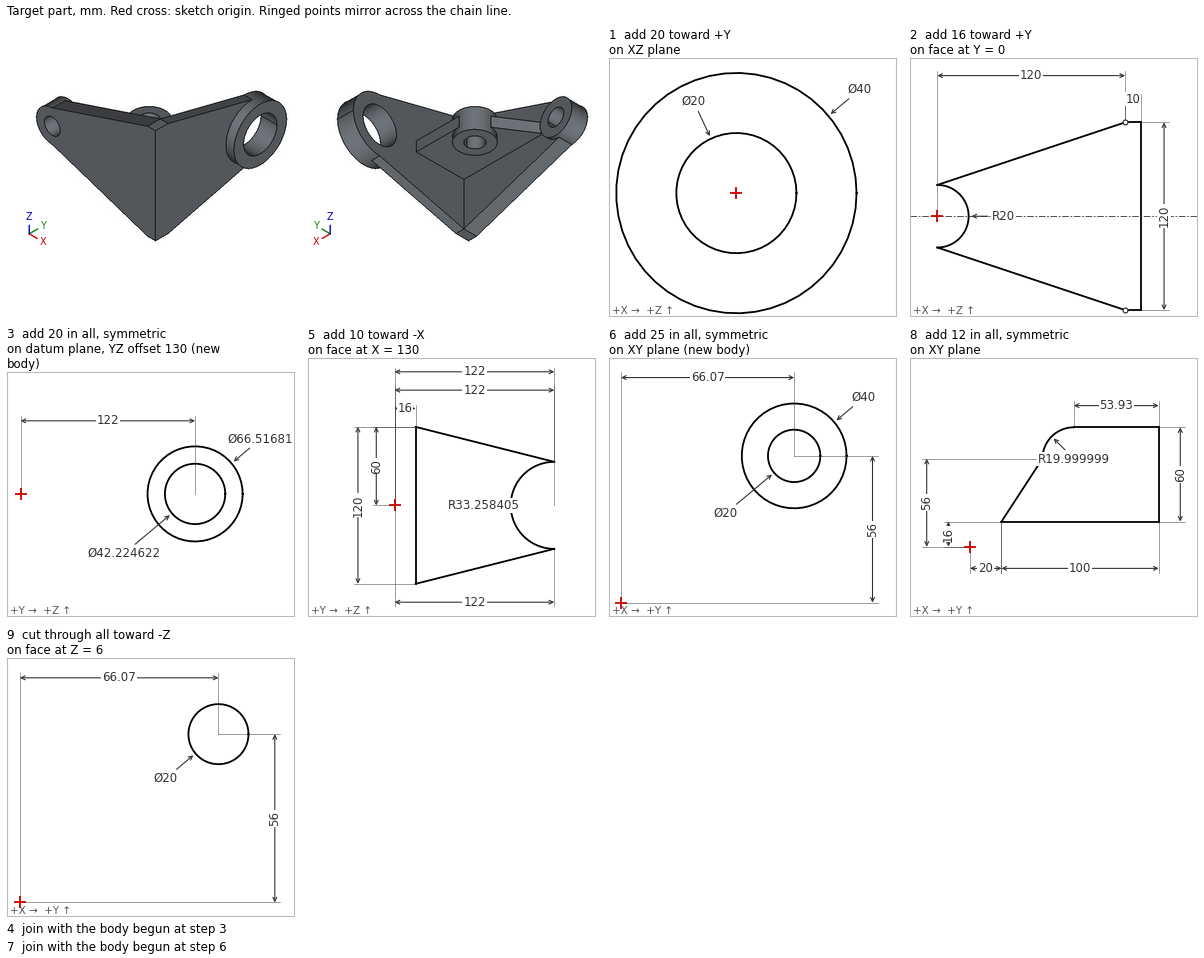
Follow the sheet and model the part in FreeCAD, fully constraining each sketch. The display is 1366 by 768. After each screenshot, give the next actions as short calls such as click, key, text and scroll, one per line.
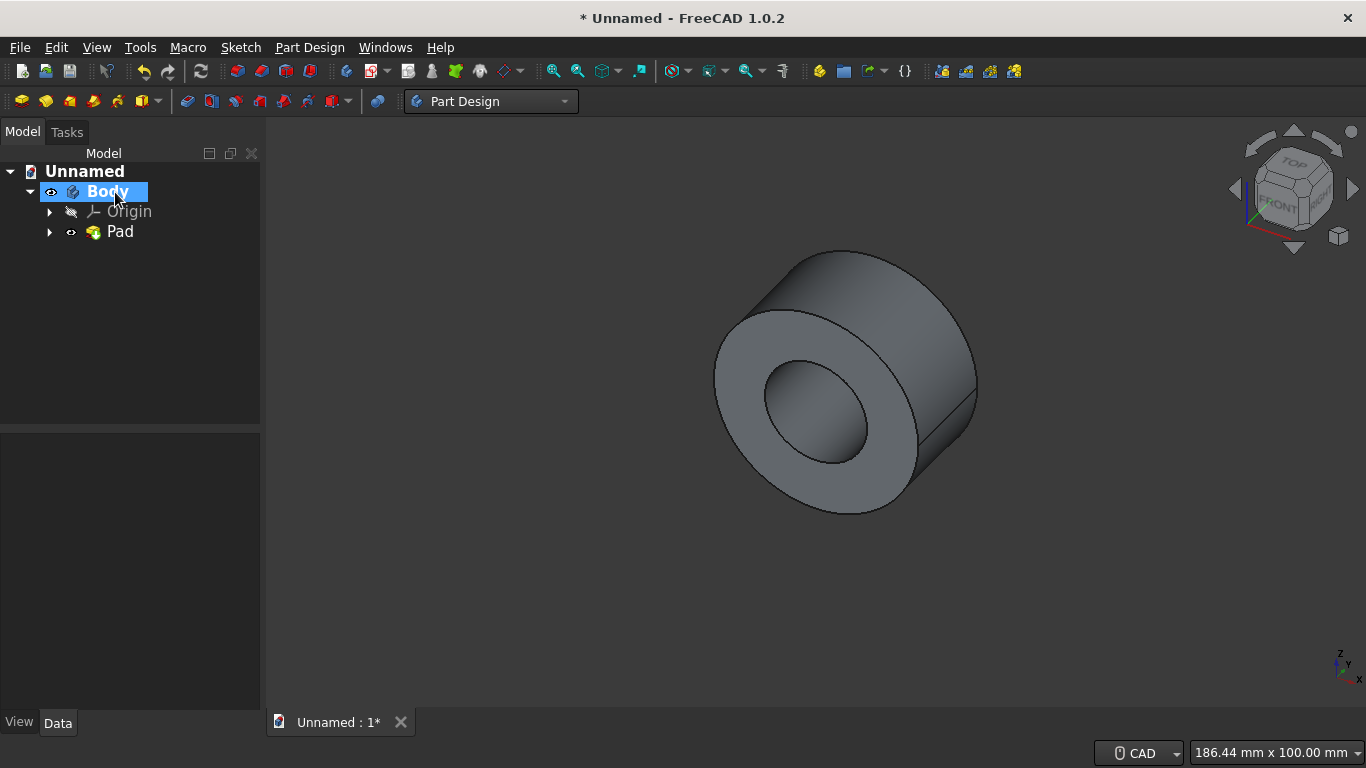
click(874, 486)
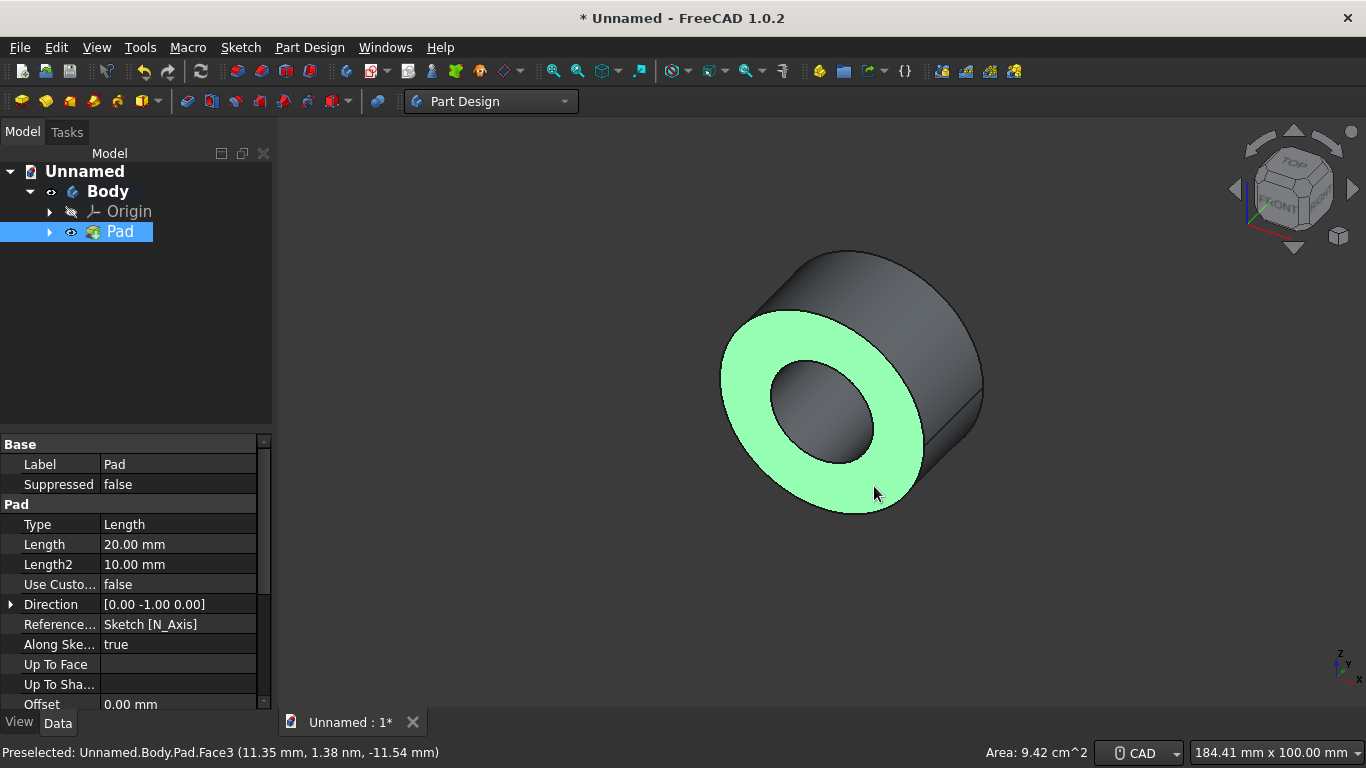
click(372, 72)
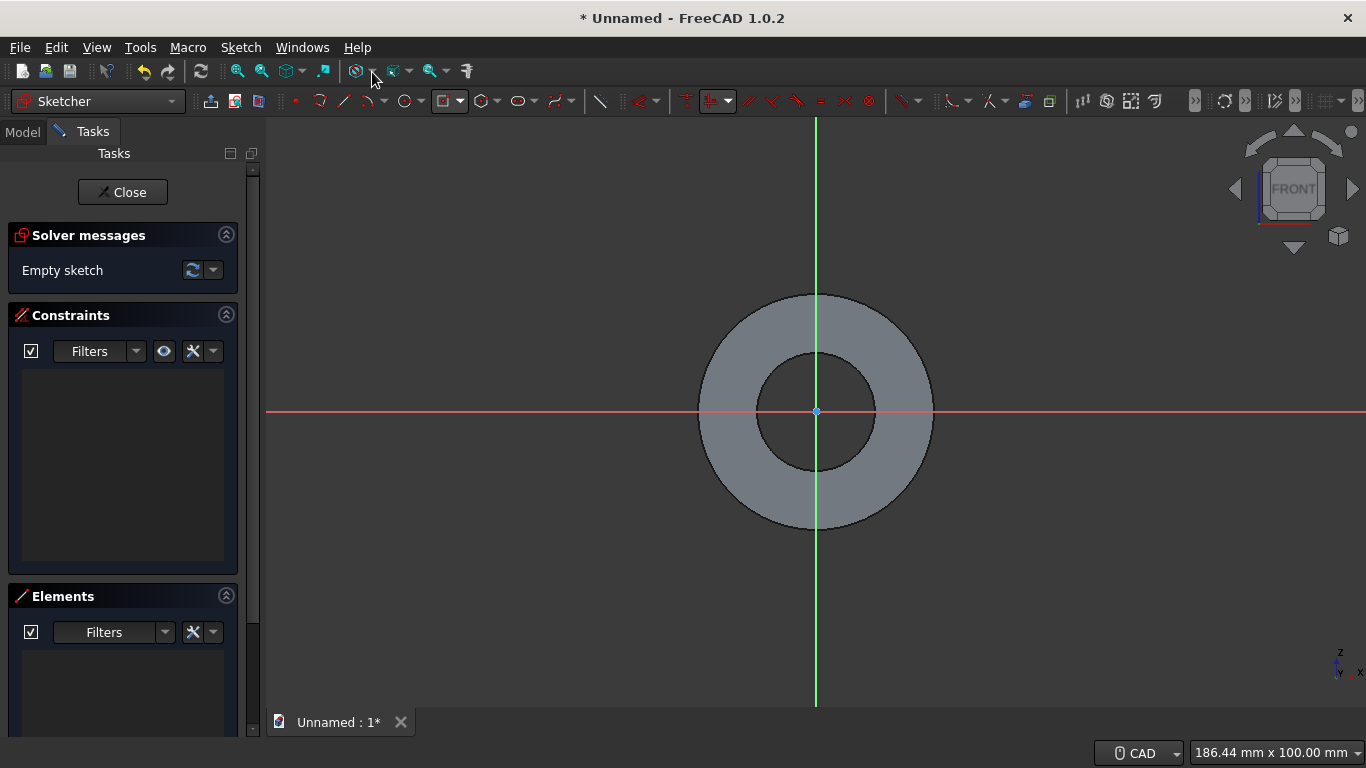
scroll(294, 412, down, 3)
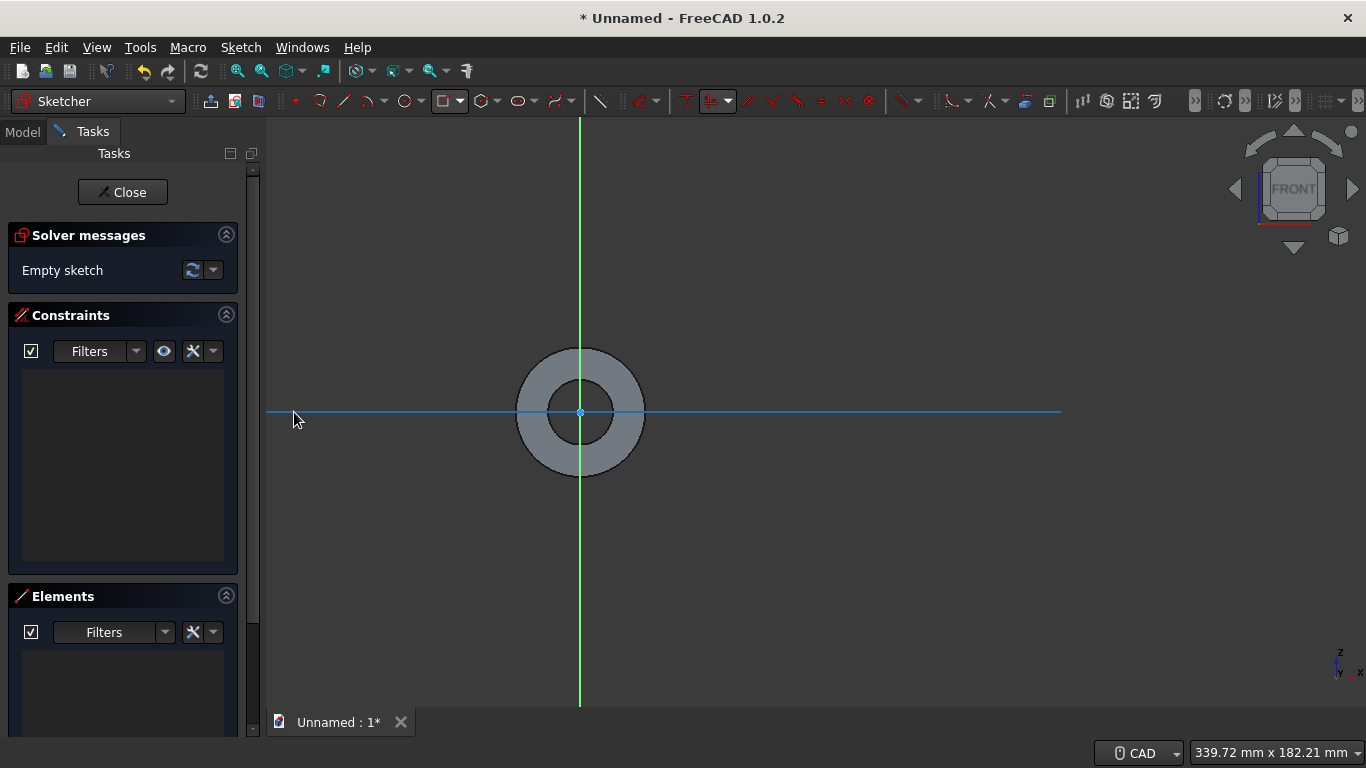
click(320, 102)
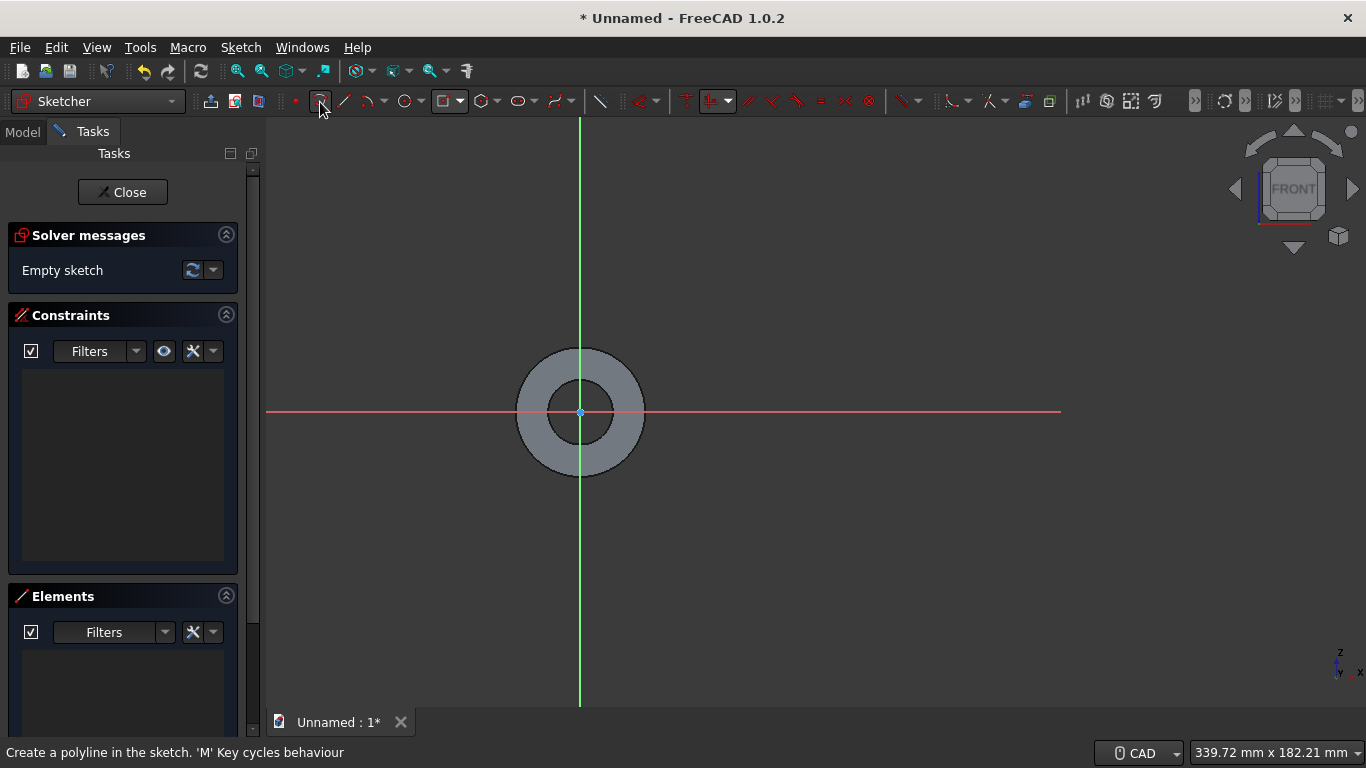
click(580, 347)
click(969, 218)
click(1001, 218)
click(1001, 607)
click(969, 607)
click(580, 477)
right_click(580, 477)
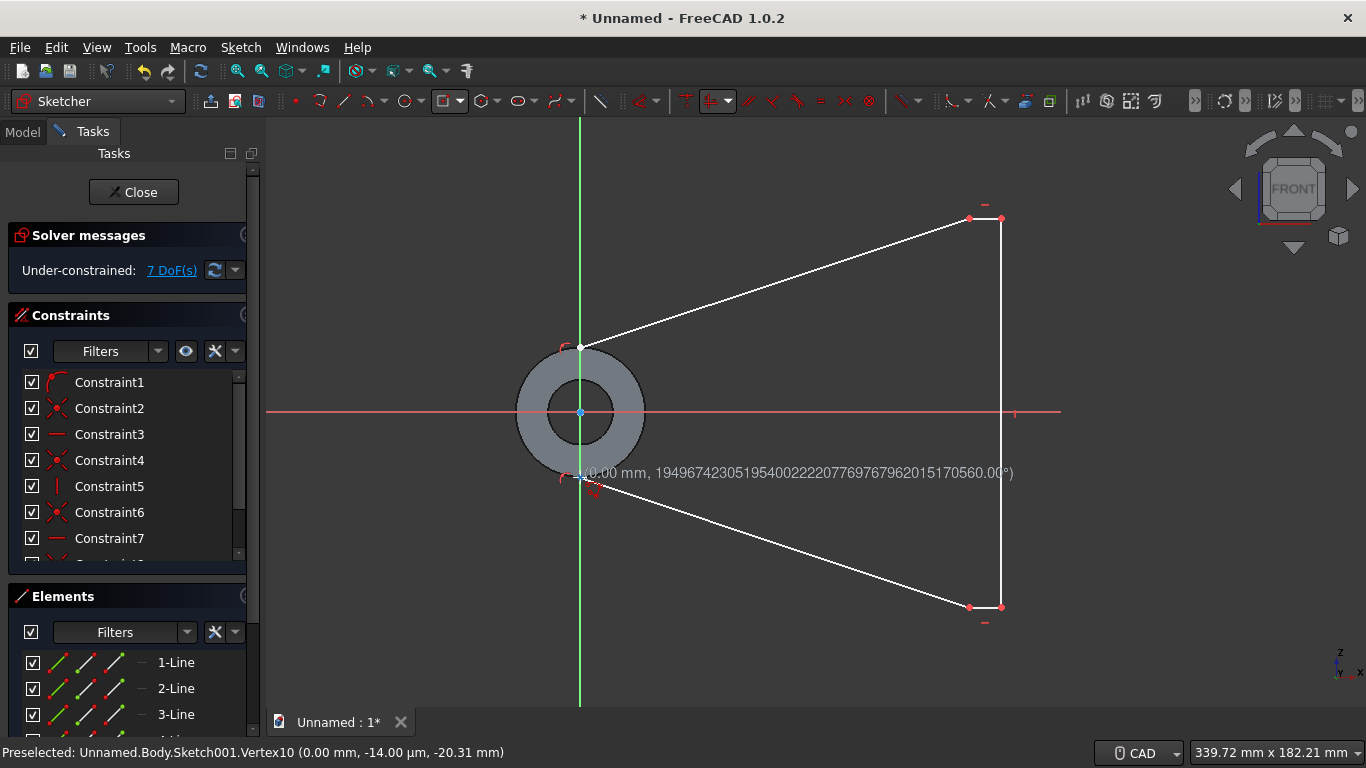
key(g)
key(3)
key(a)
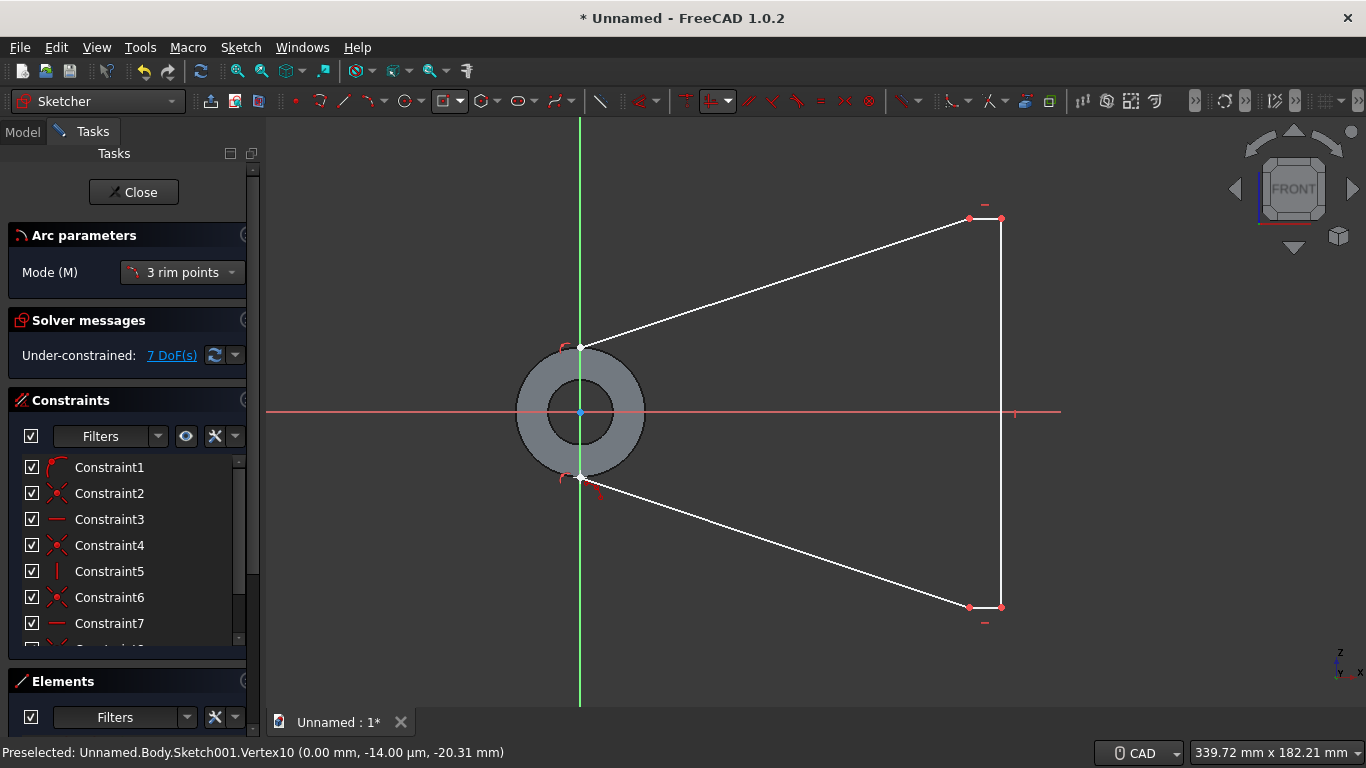
click(580, 478)
click(580, 348)
click(642, 432)
key(Escape)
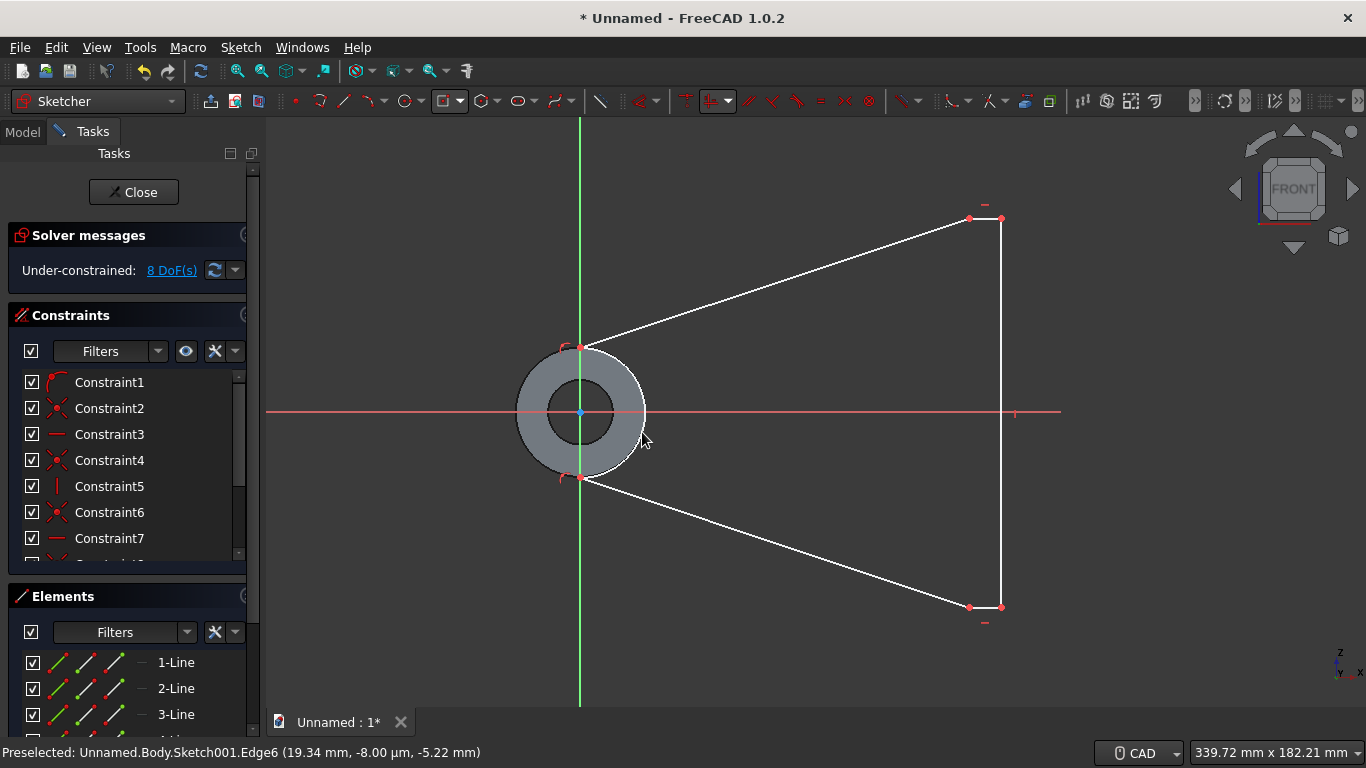
drag(570, 402, 590, 423)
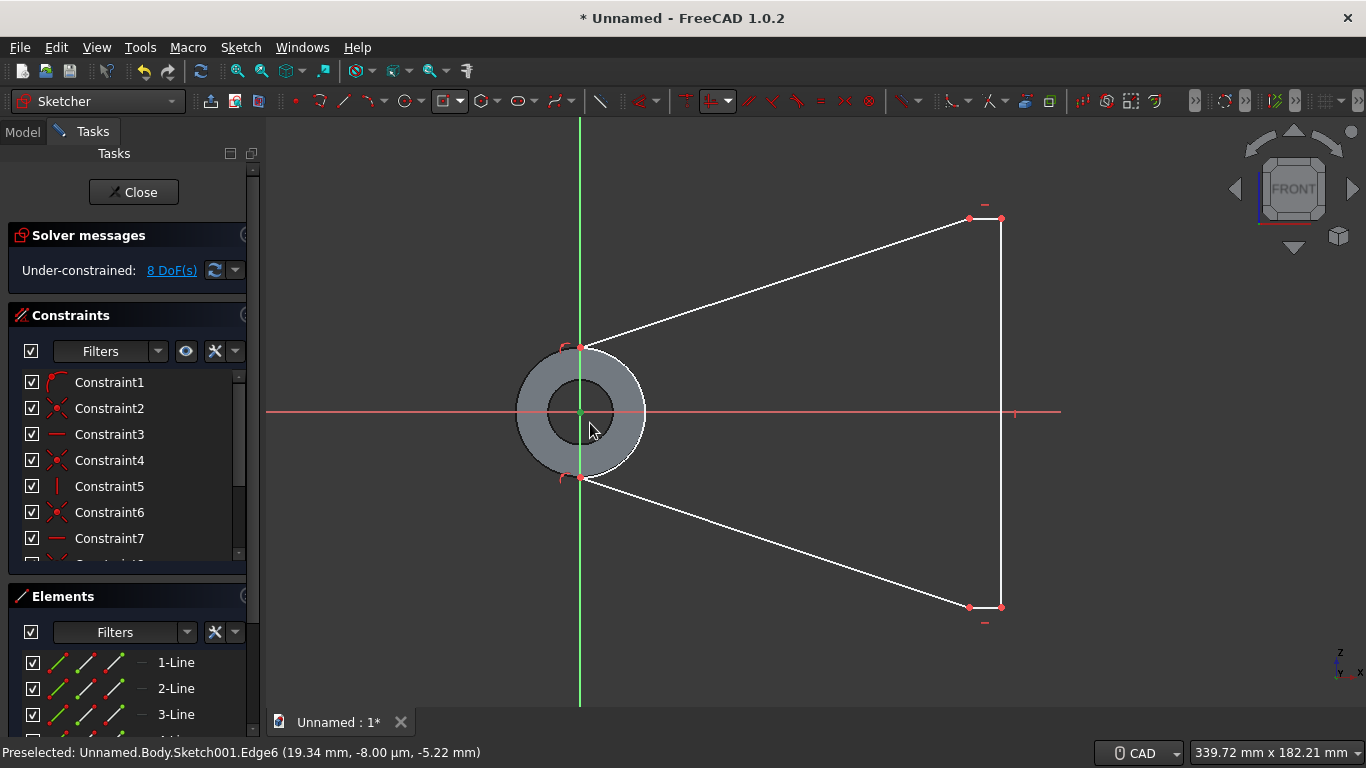
click(686, 102)